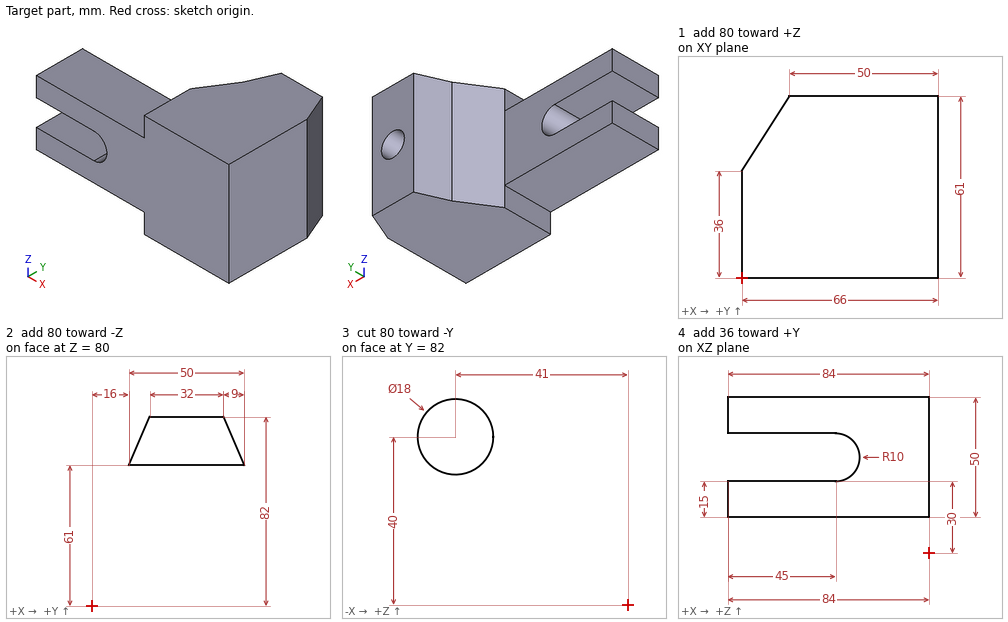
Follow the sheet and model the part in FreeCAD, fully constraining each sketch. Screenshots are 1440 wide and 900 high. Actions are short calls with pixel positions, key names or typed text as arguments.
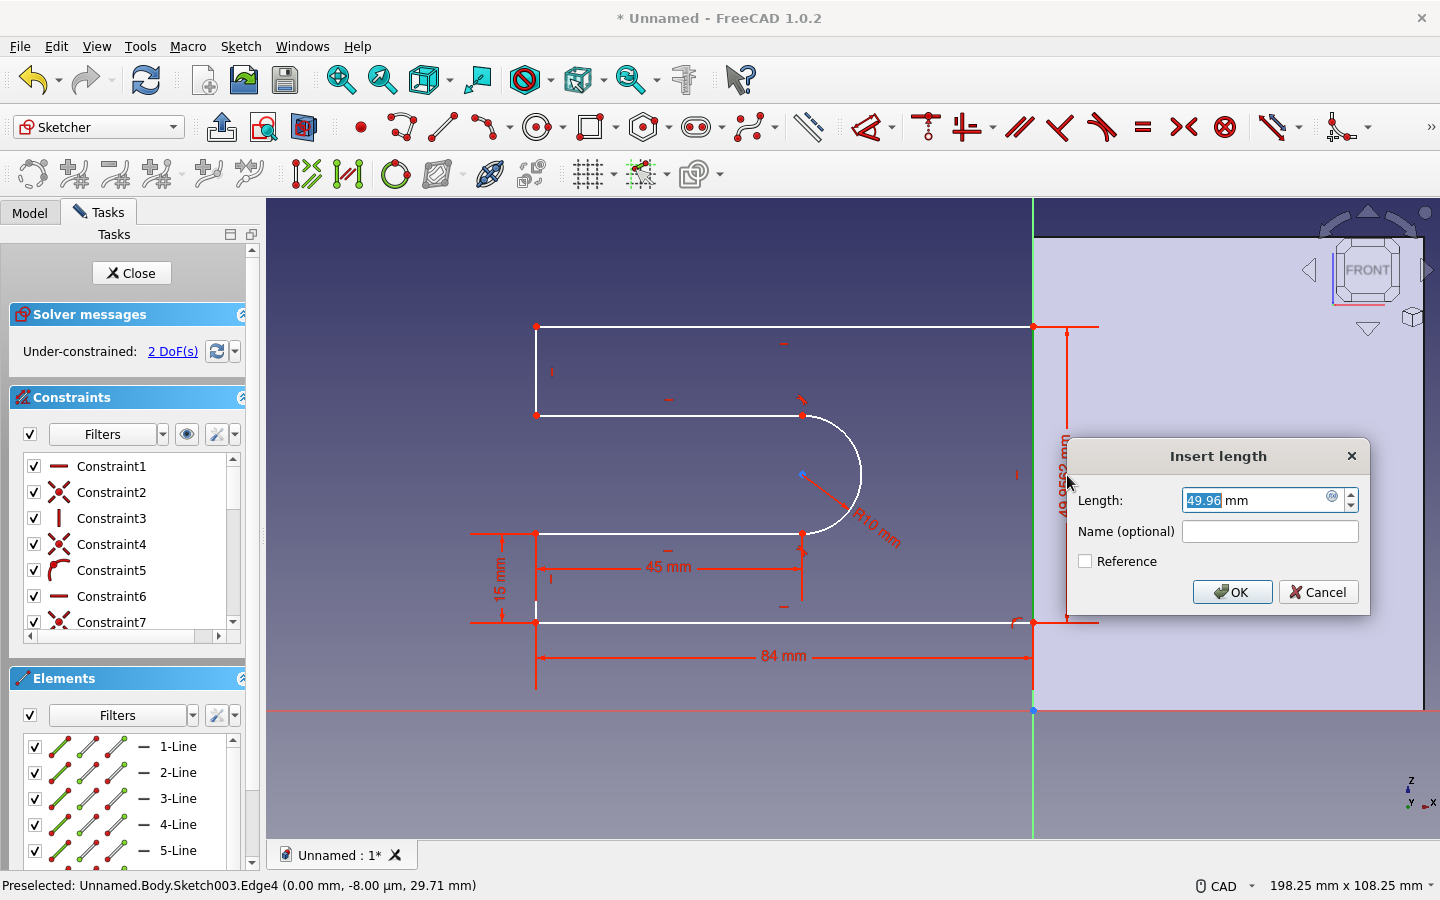
text(50)
key(Return)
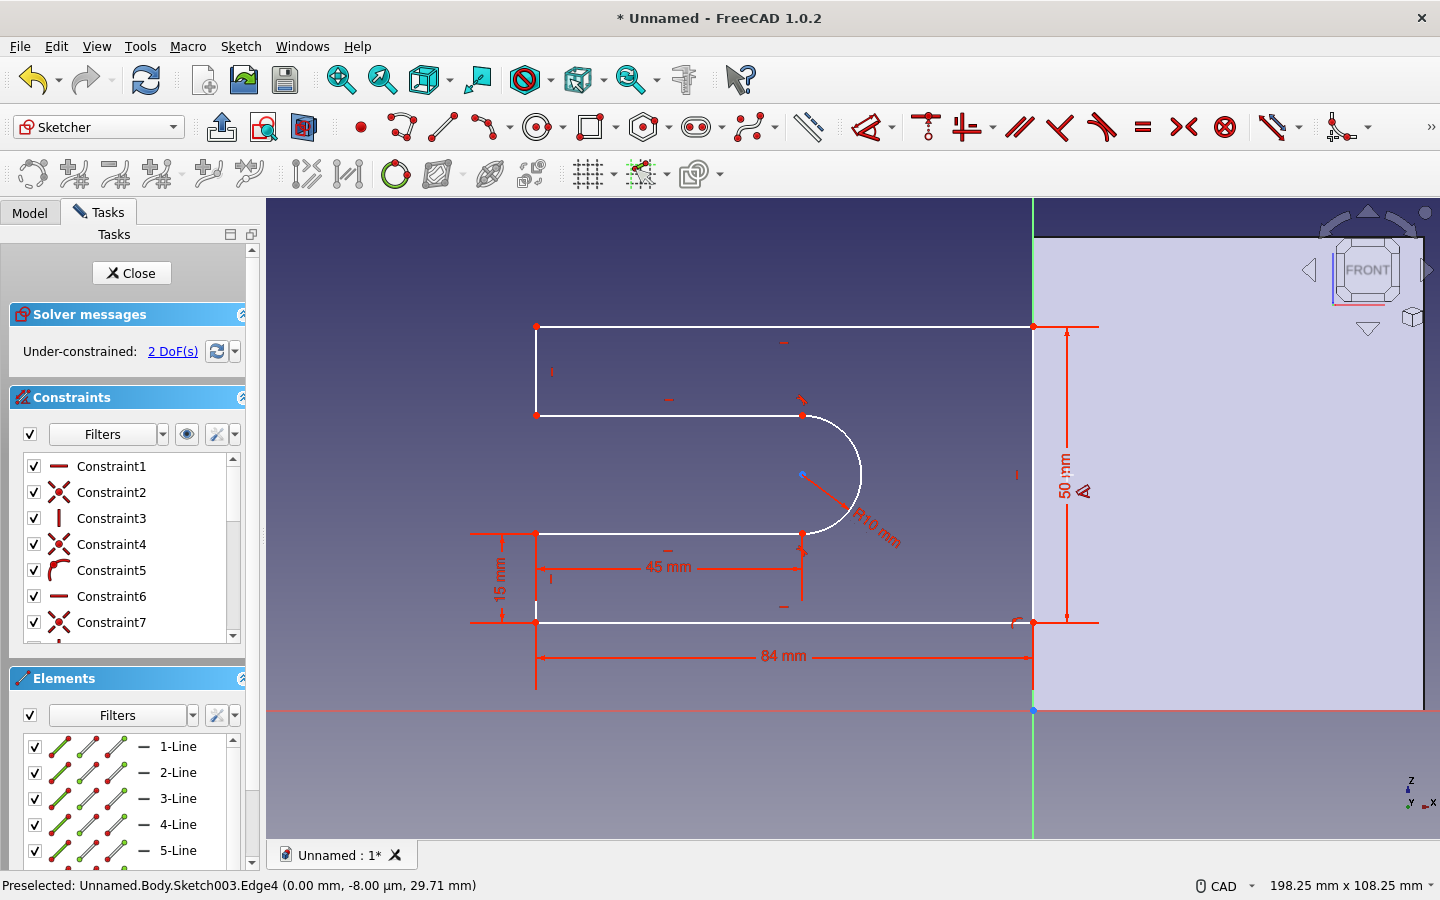
click(884, 327)
click(785, 293)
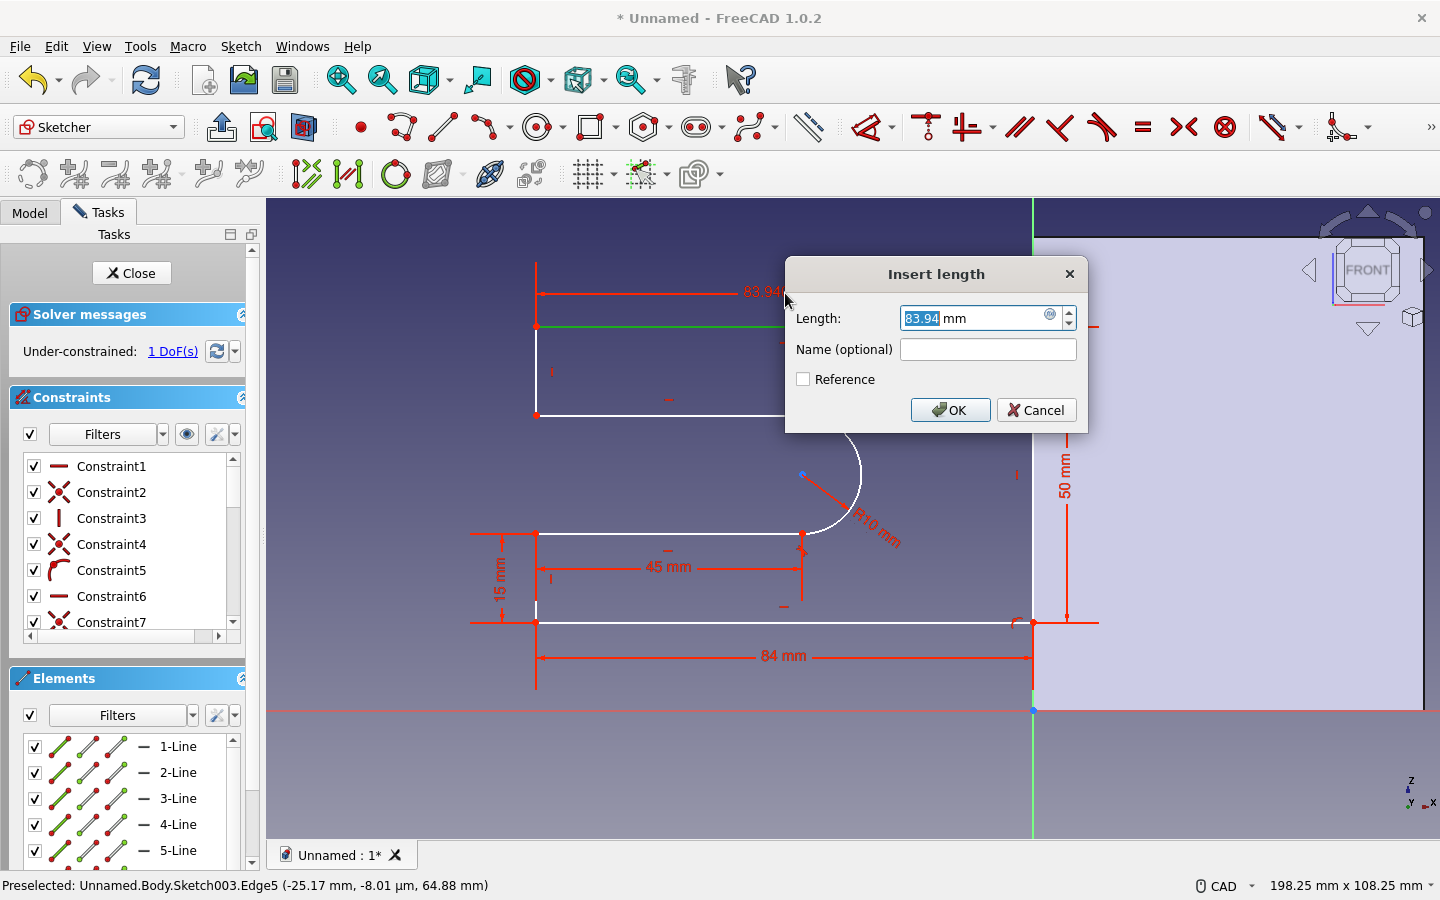
text(84)
key(Return)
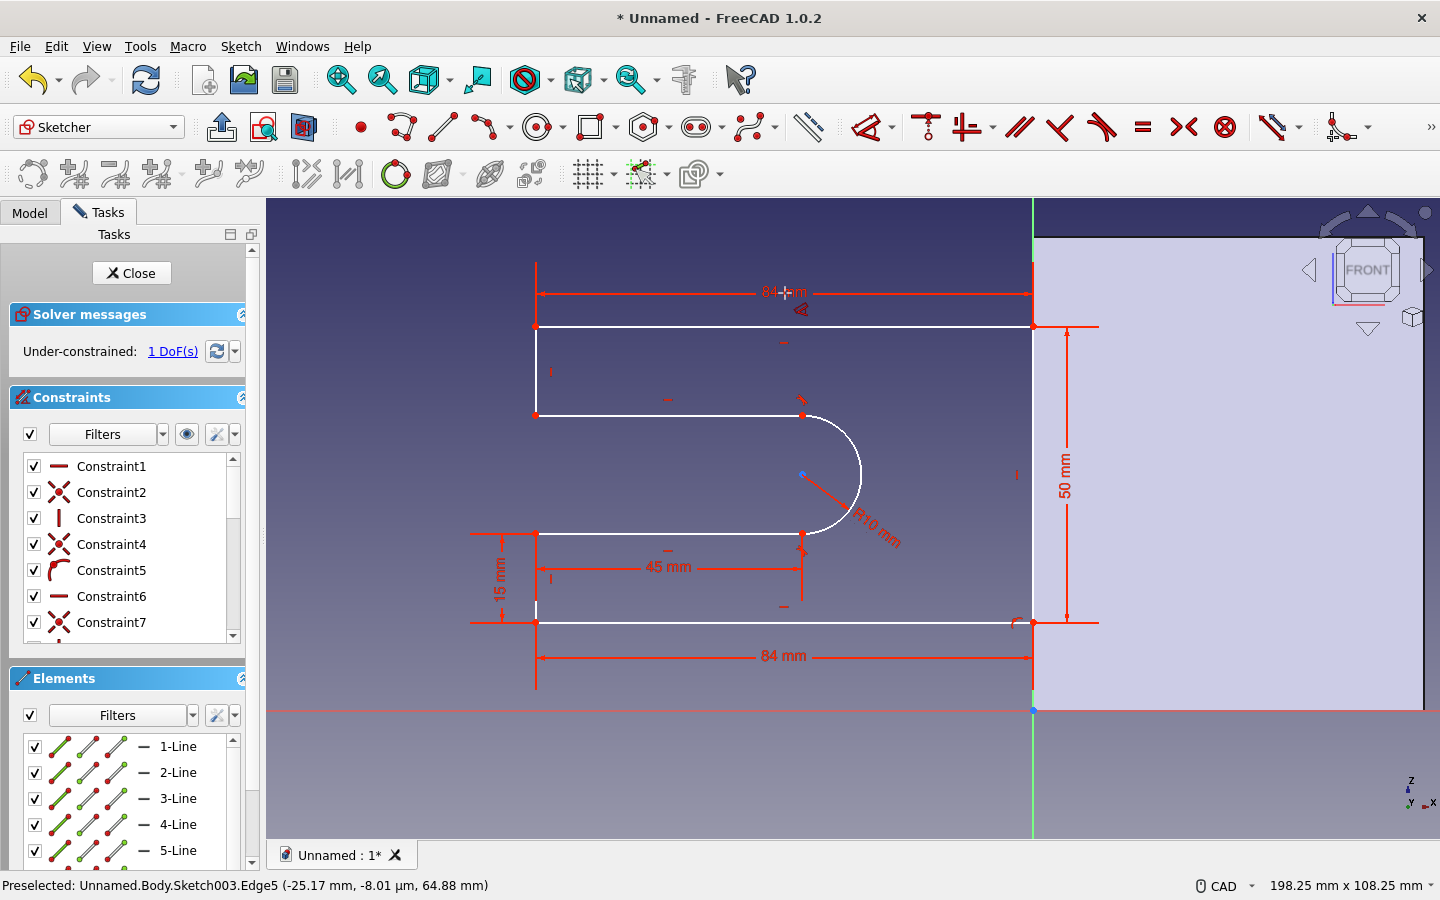
click(802, 534)
click(1067, 622)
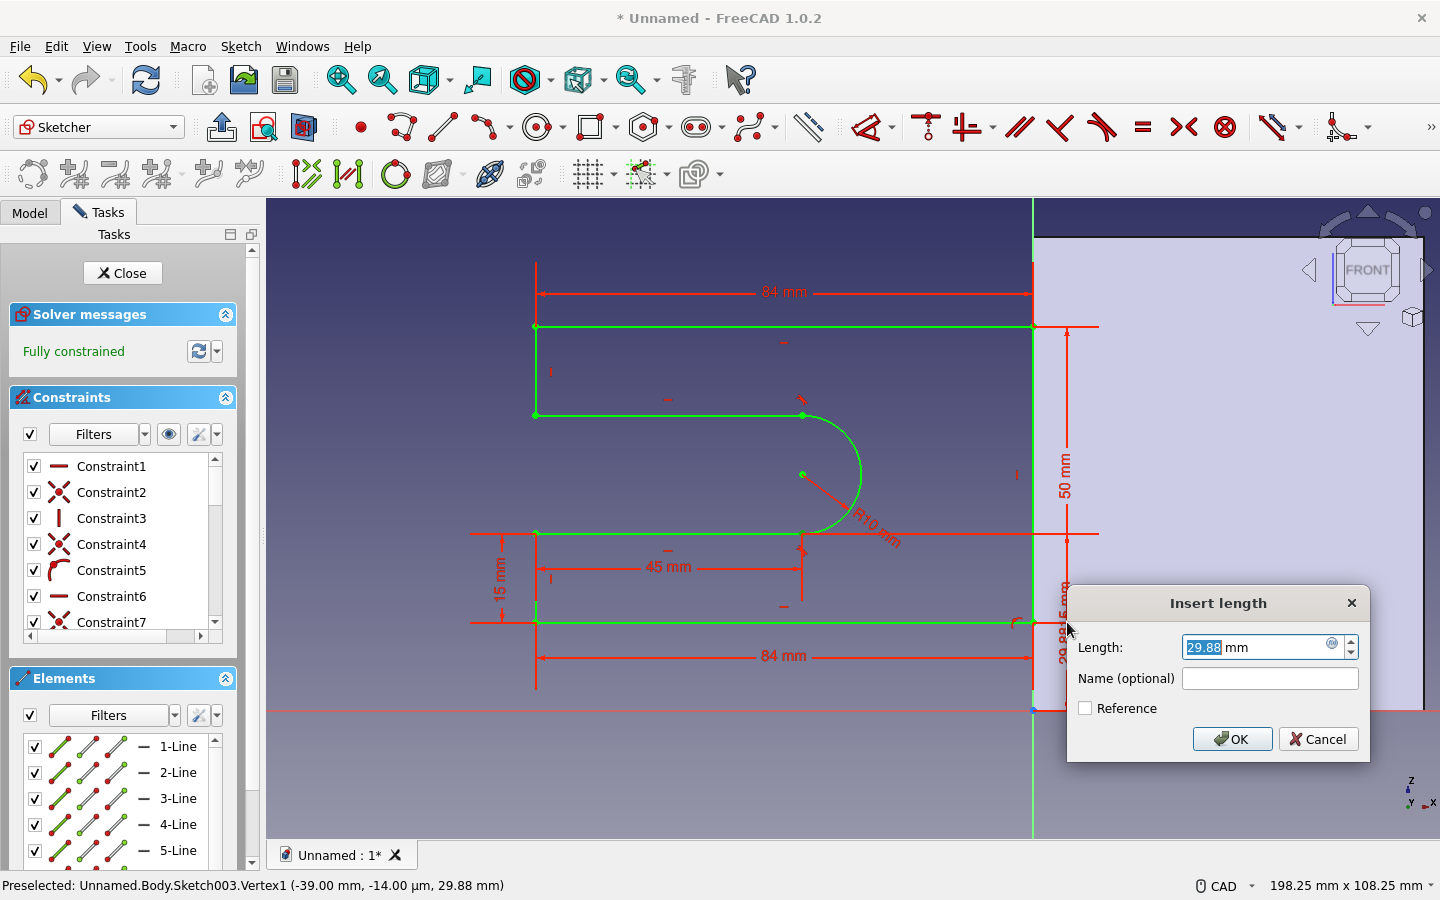
text(30)
key(Return)
key(Escape)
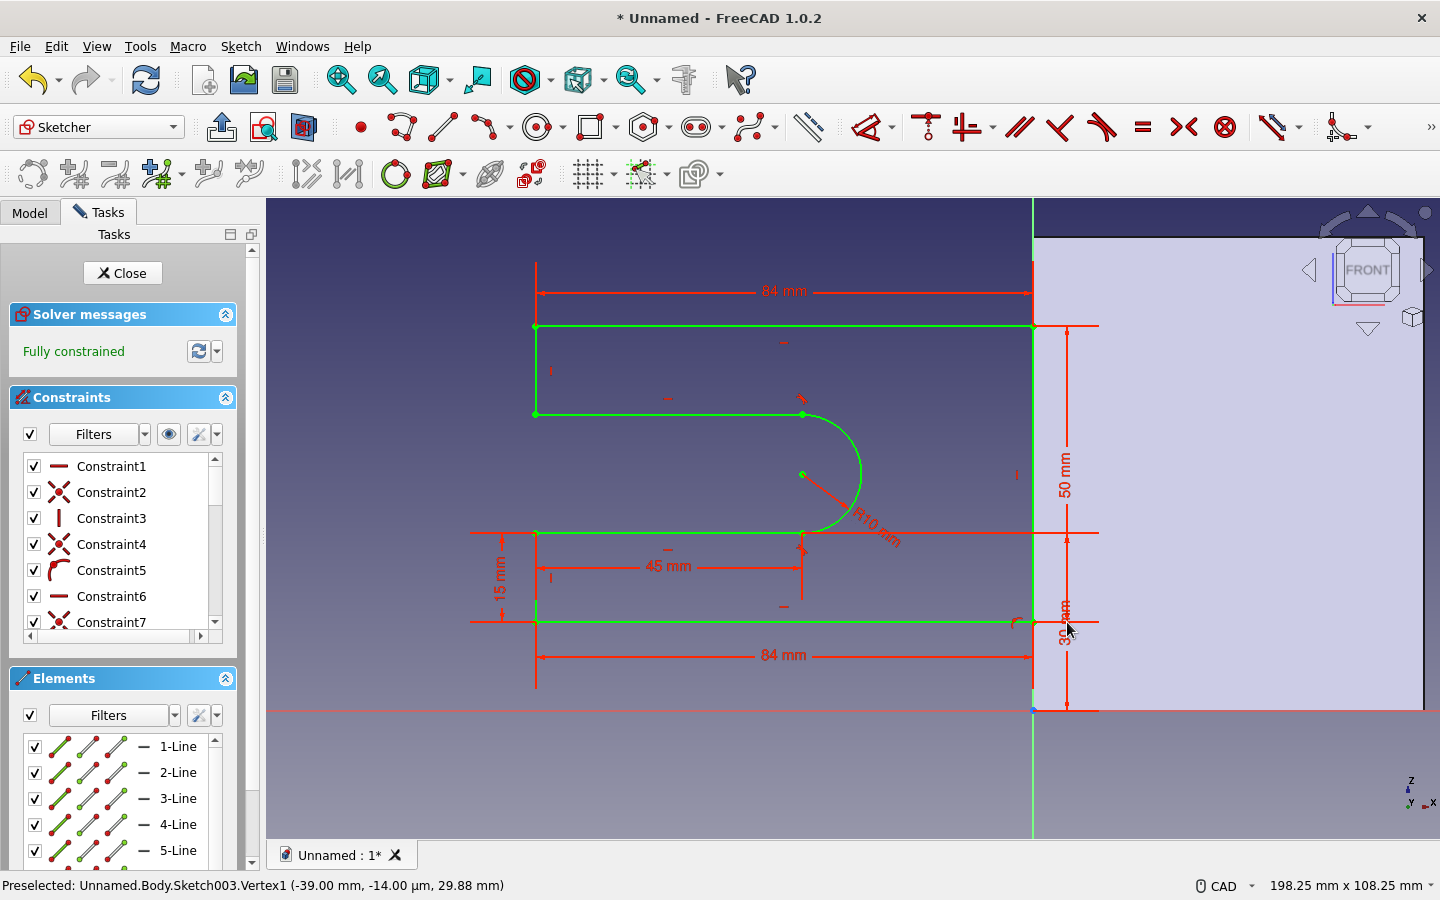
click(123, 273)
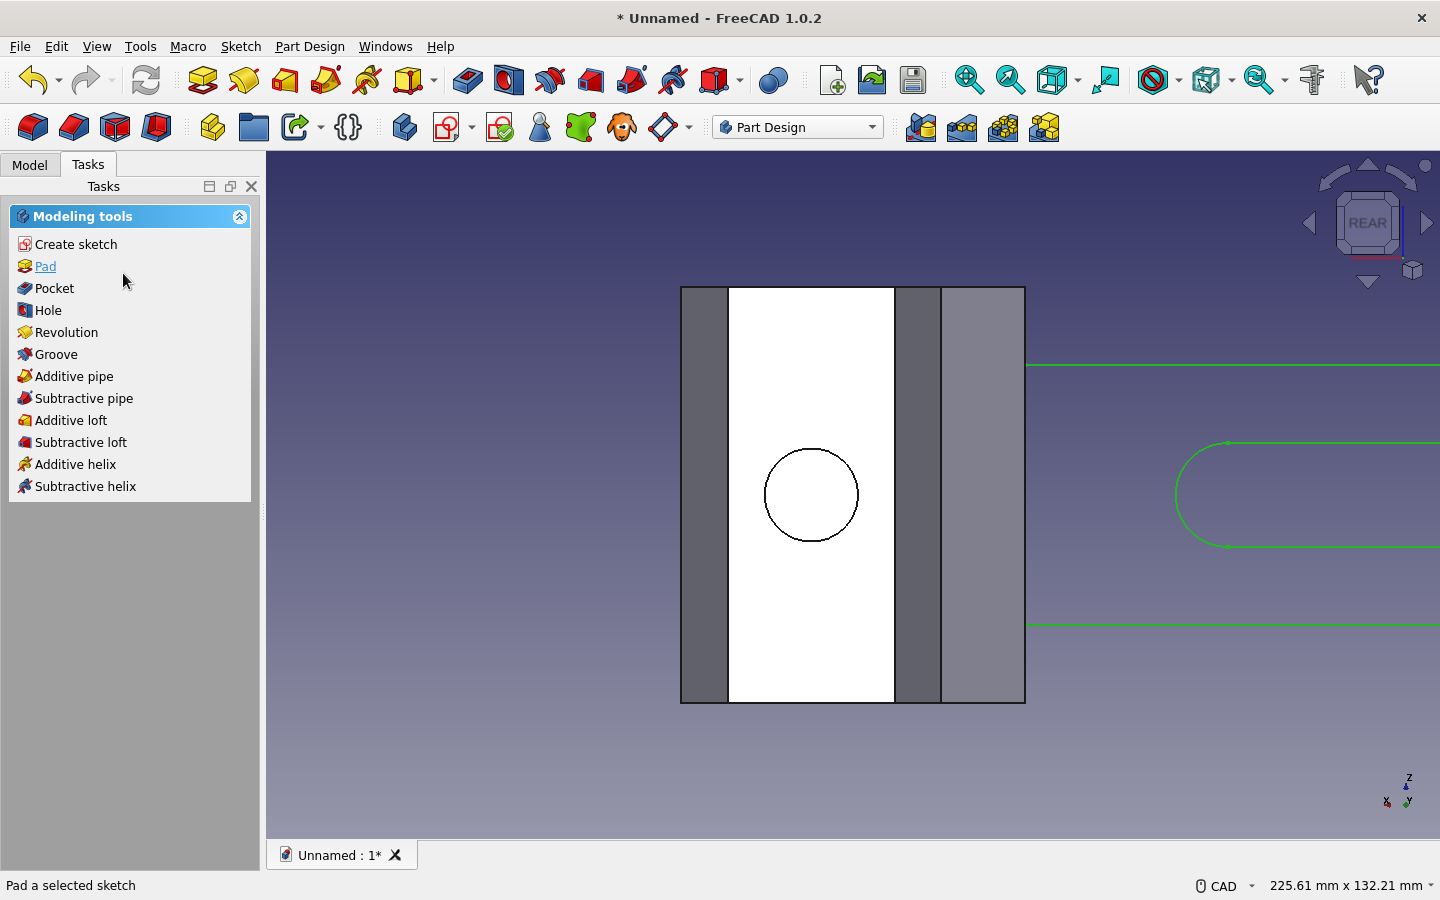
click(203, 80)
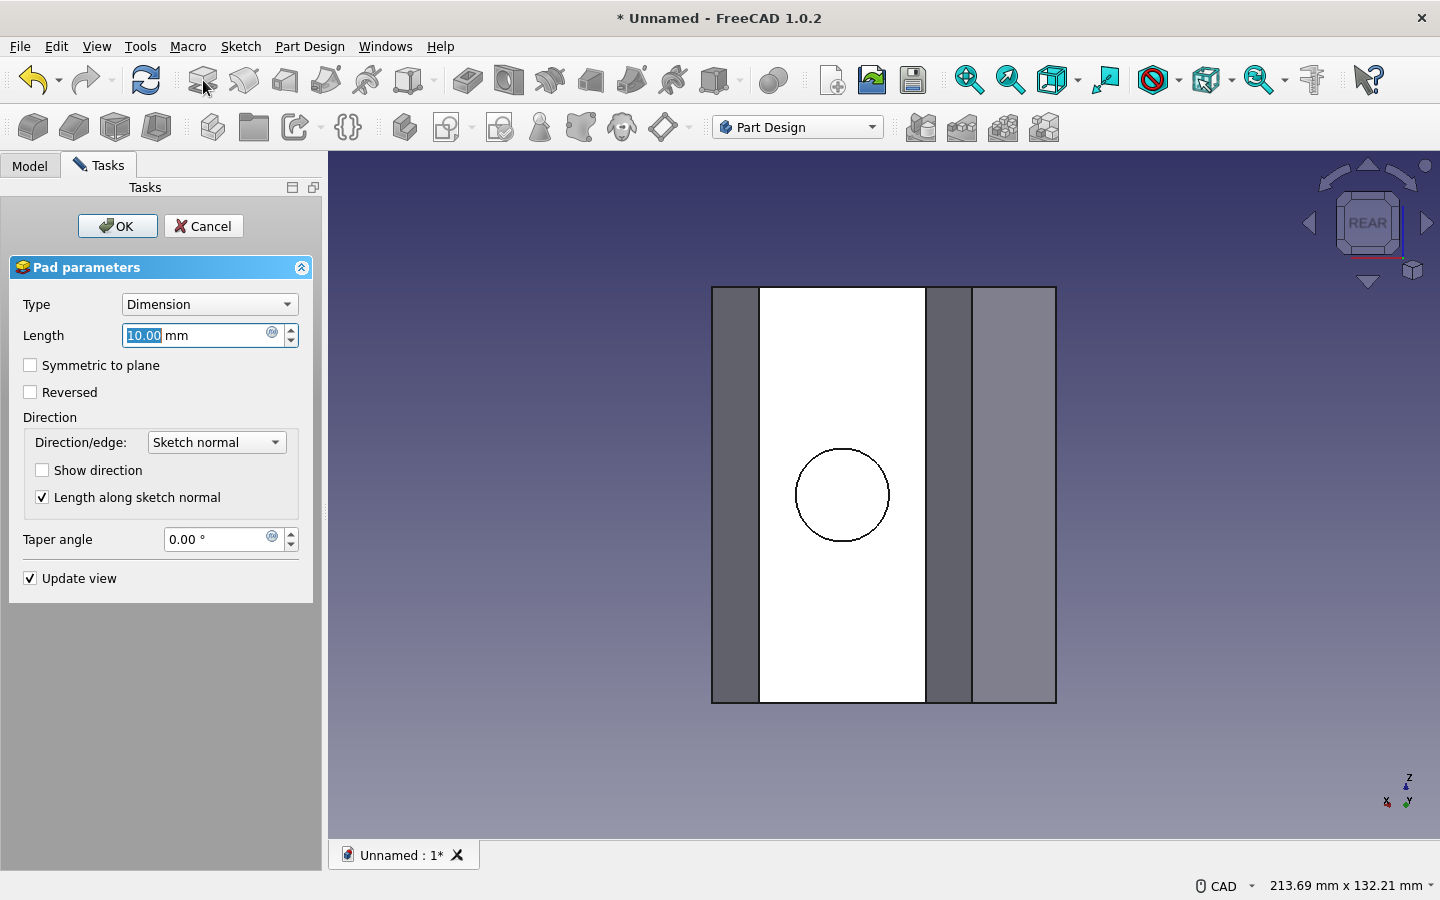
text(36)
key(Tab)